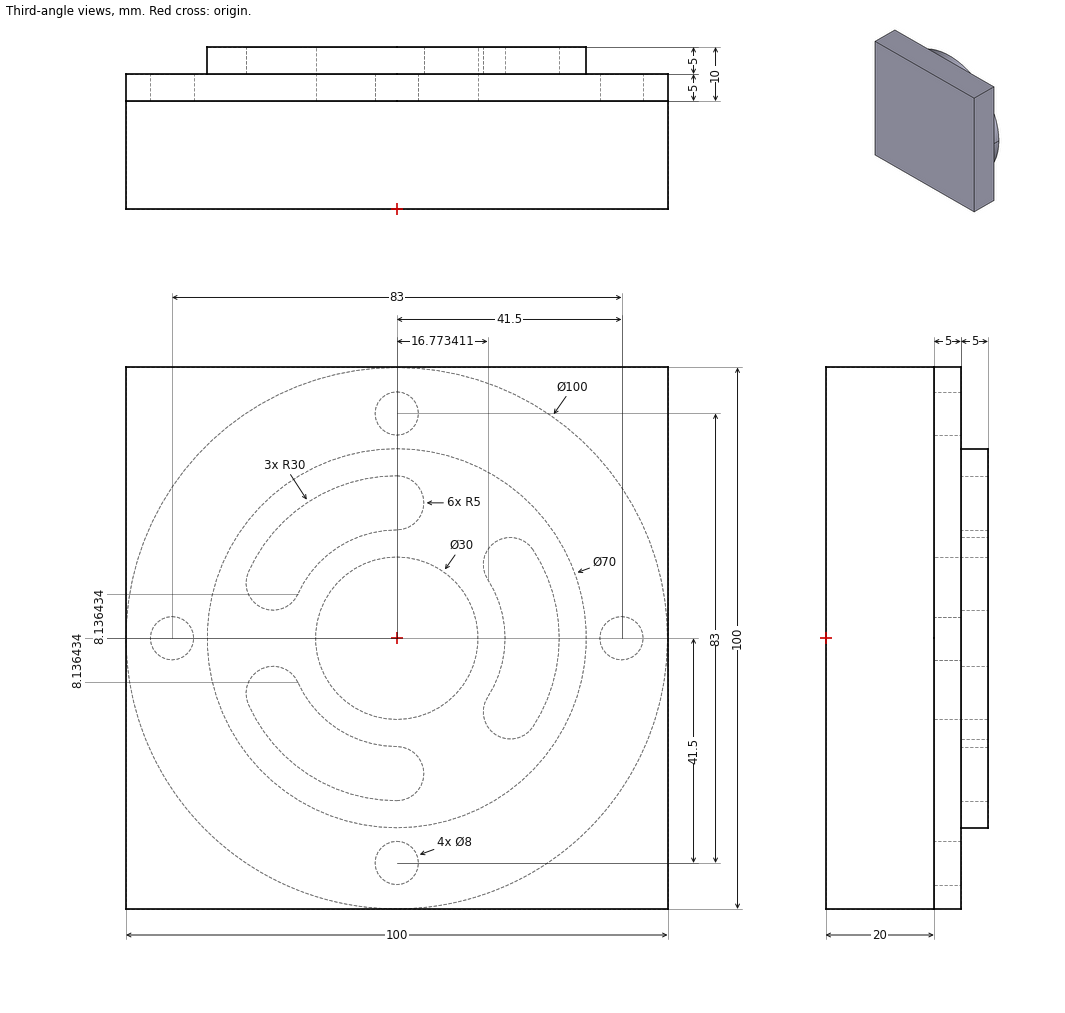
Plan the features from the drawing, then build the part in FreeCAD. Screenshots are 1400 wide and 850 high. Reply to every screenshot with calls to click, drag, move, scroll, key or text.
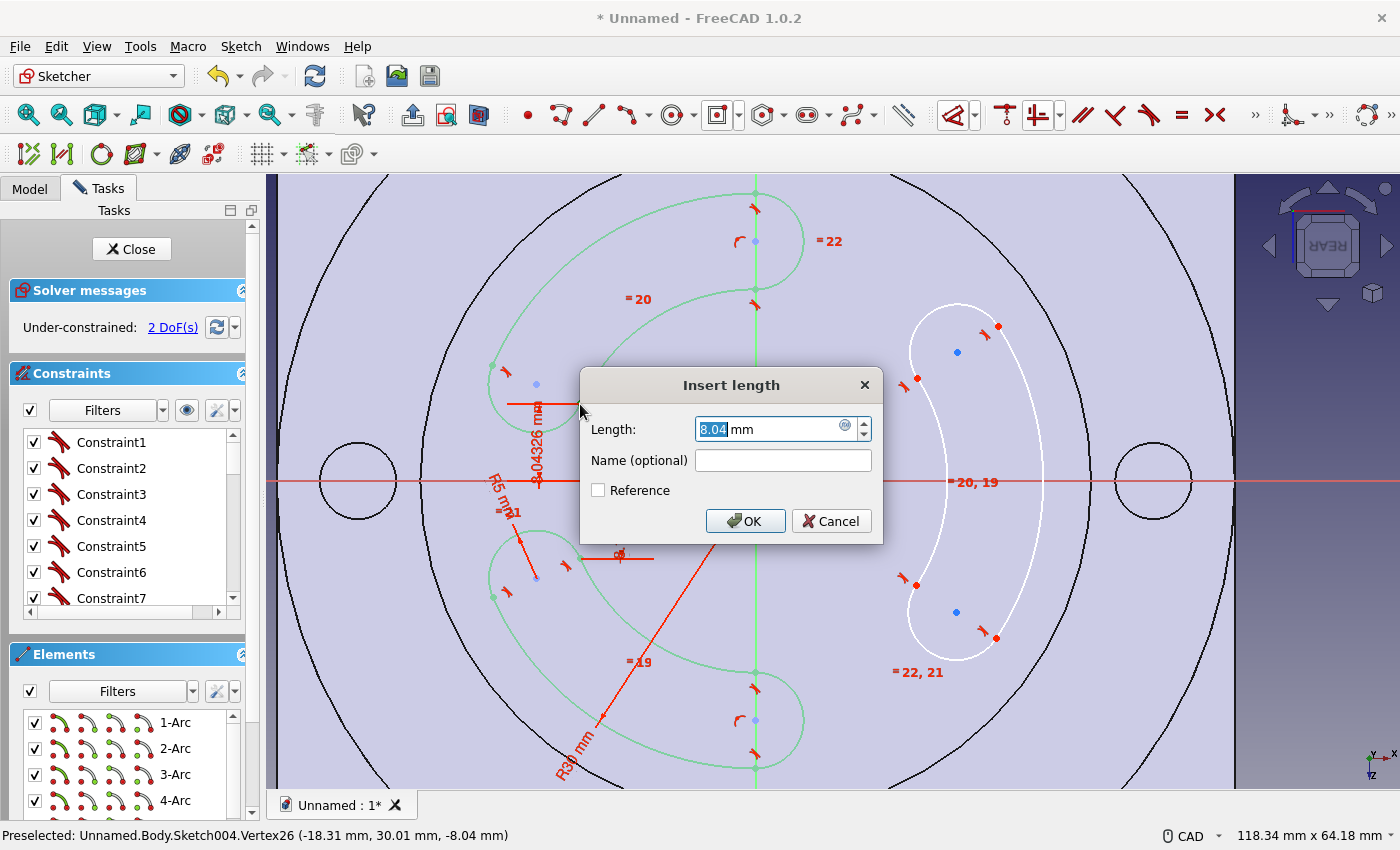
text(8.136434)
key(Return)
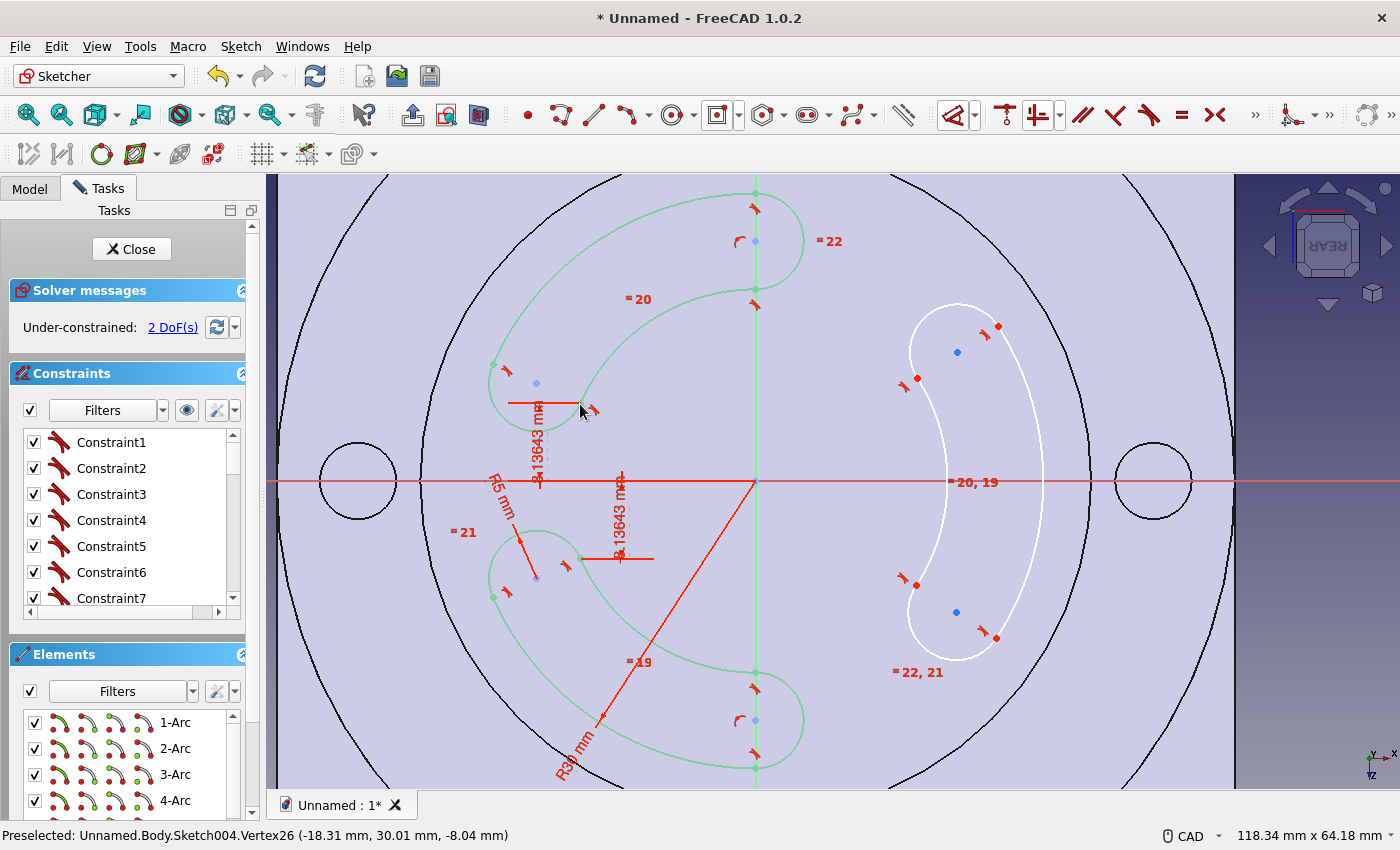
click(916, 586)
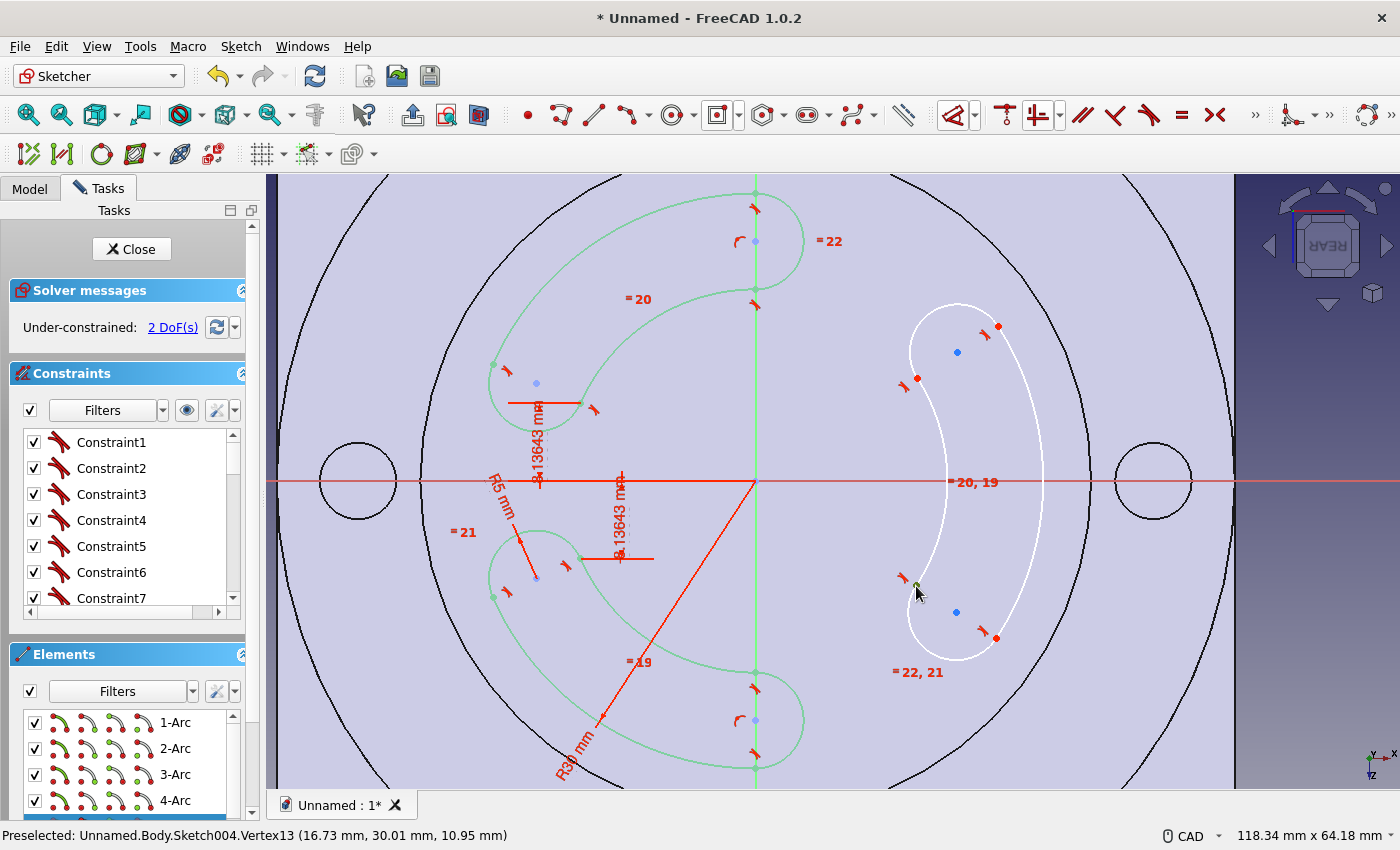
click(974, 116)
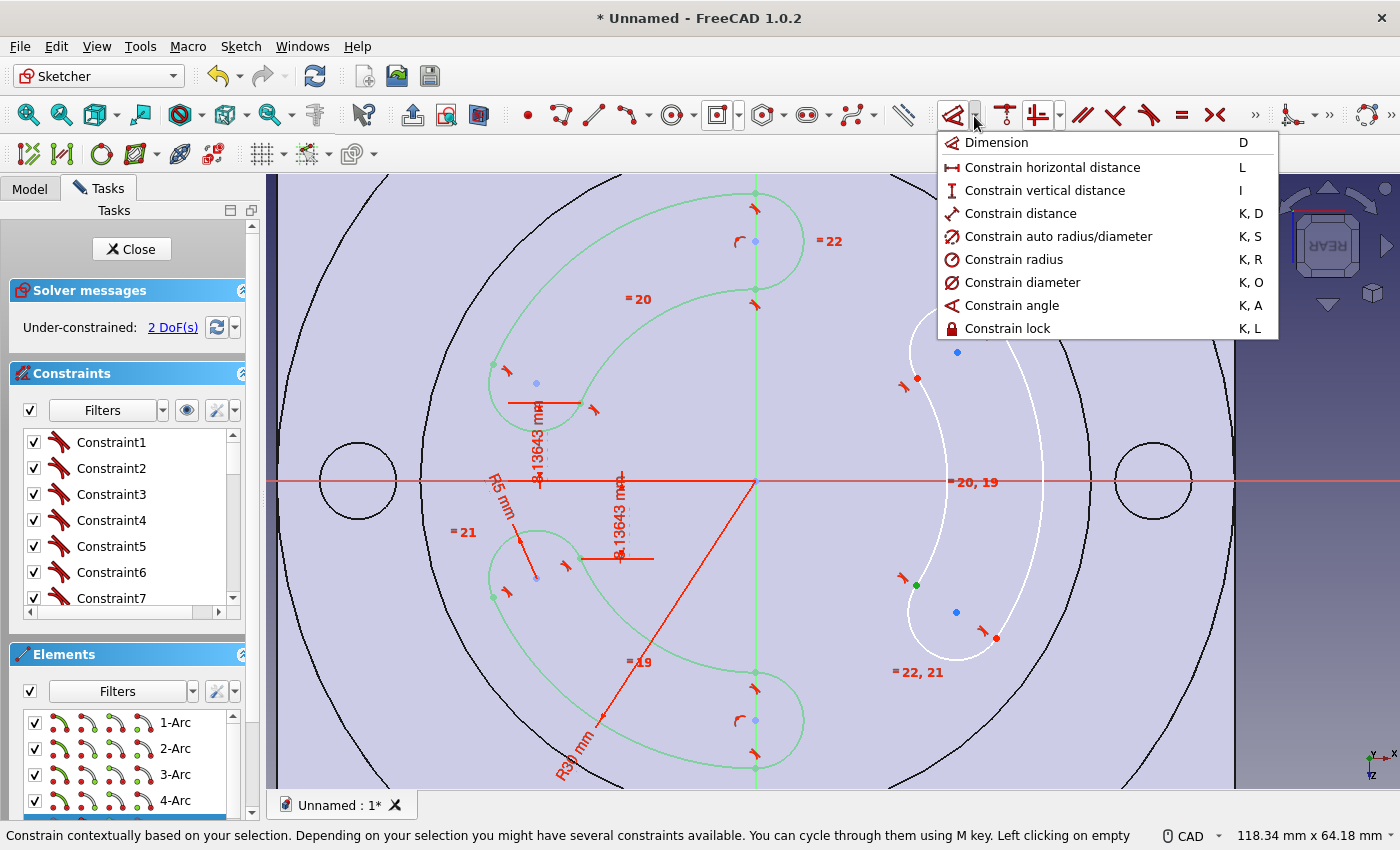
click(1108, 168)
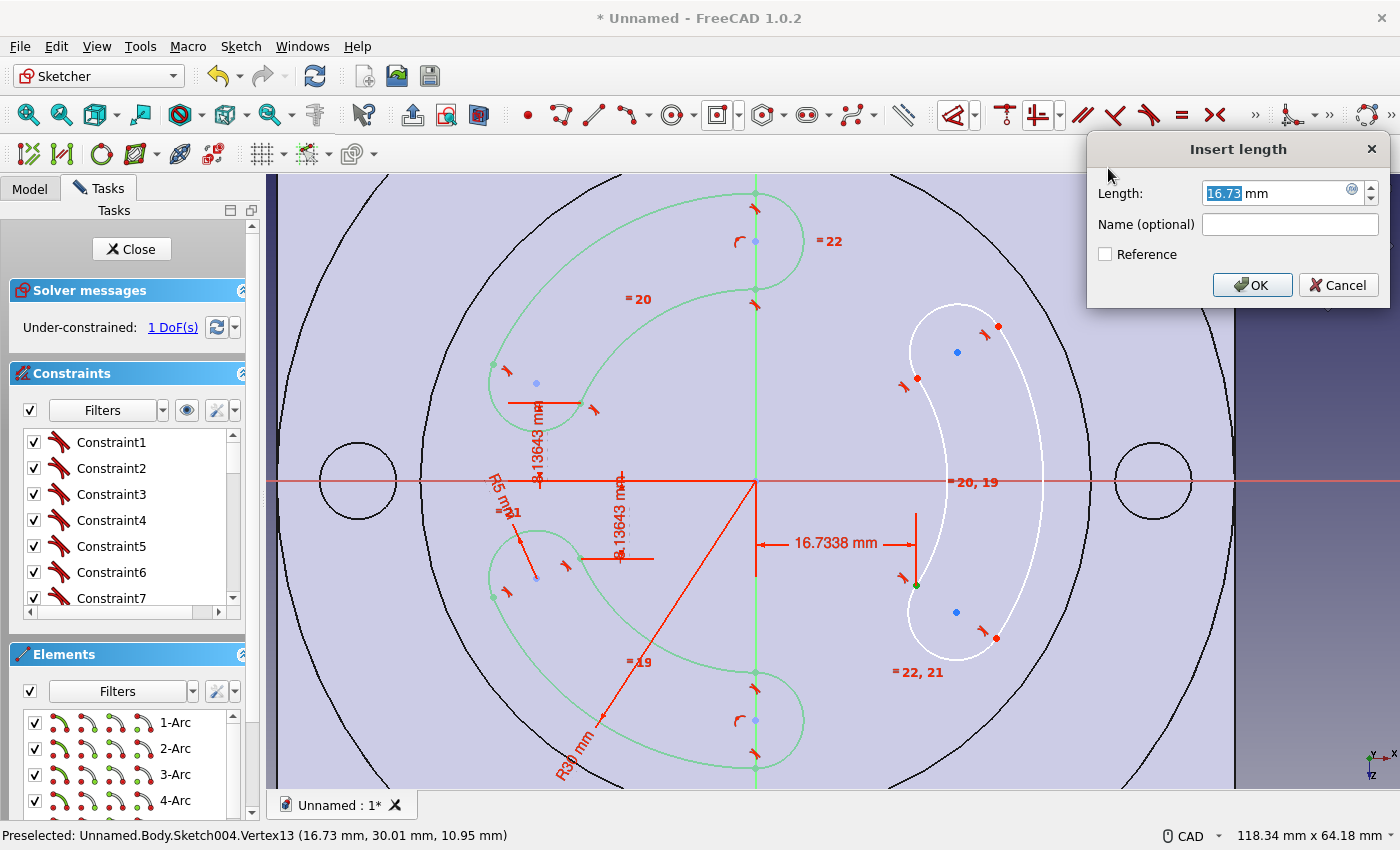
text(16.773411)
key(Return)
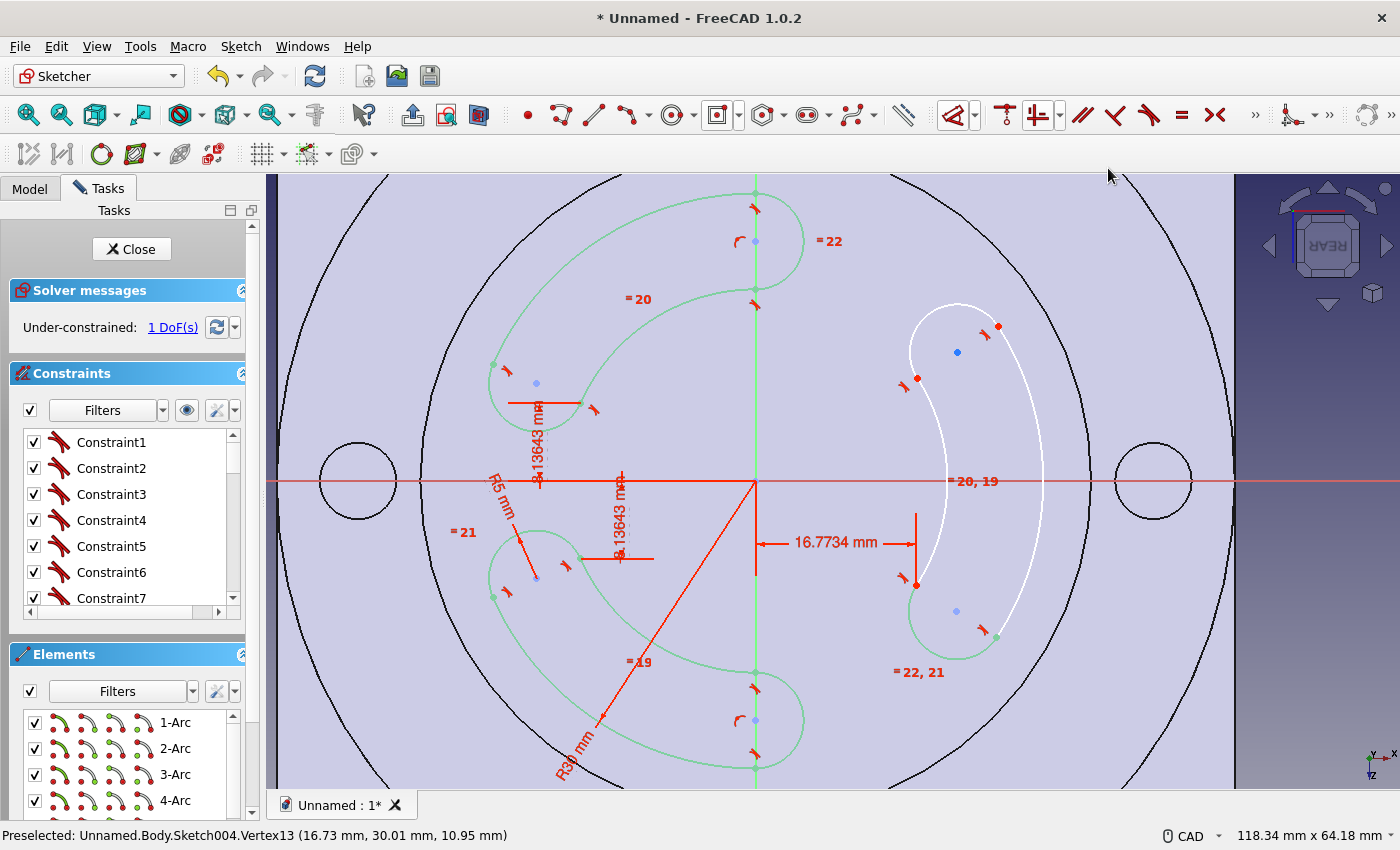
click(917, 378)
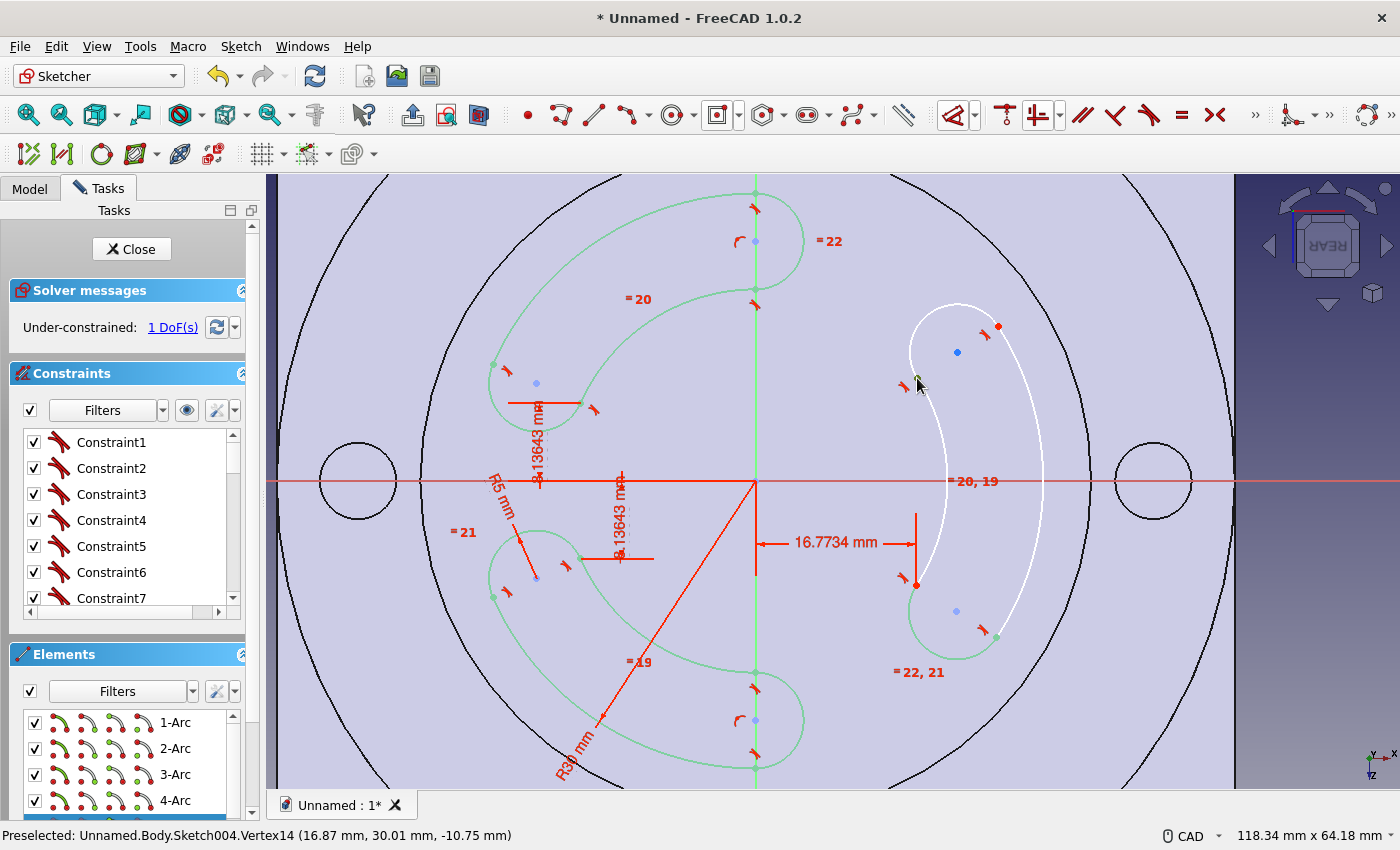
click(974, 116)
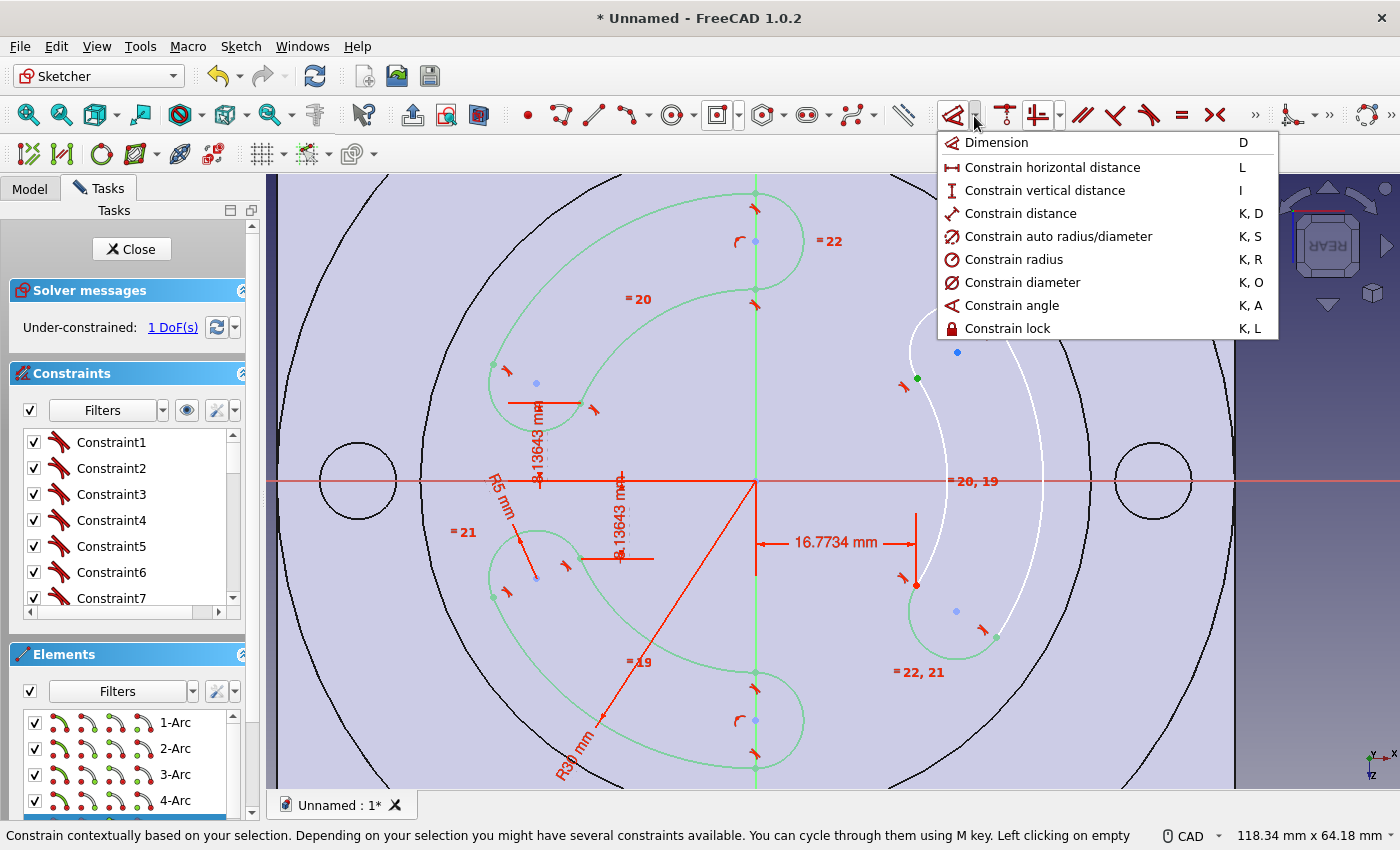
click(1108, 168)